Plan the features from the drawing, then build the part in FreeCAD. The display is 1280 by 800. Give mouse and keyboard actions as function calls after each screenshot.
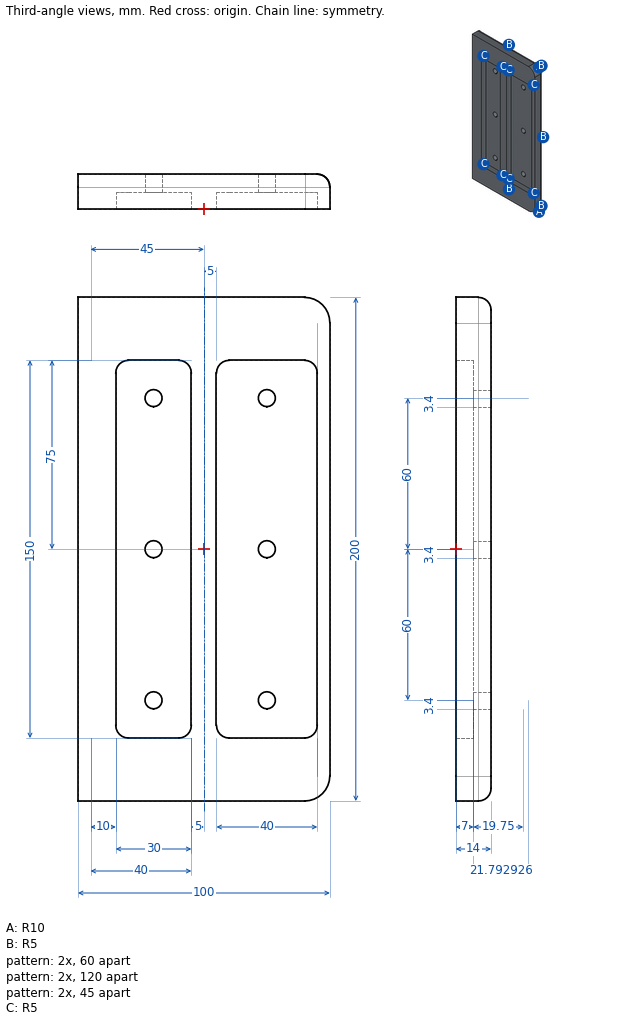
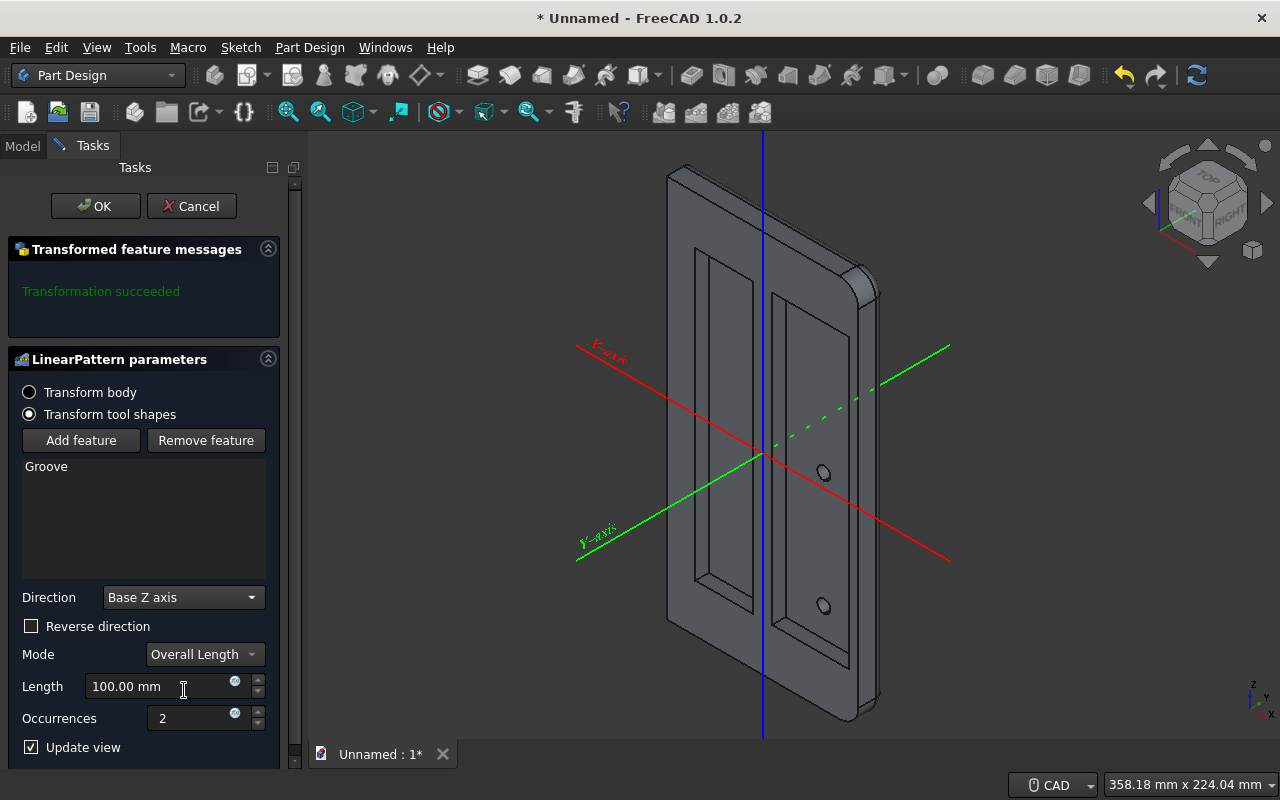
click(206, 654)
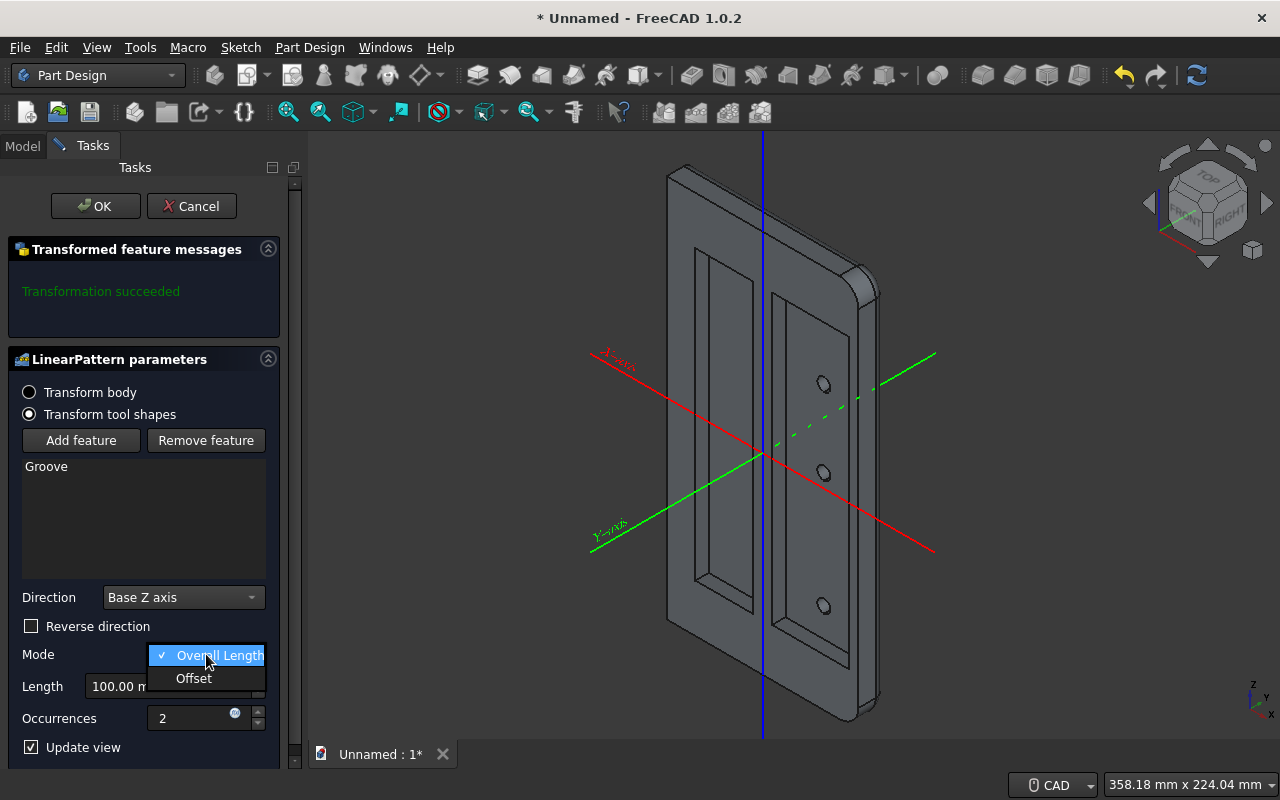
click(206, 678)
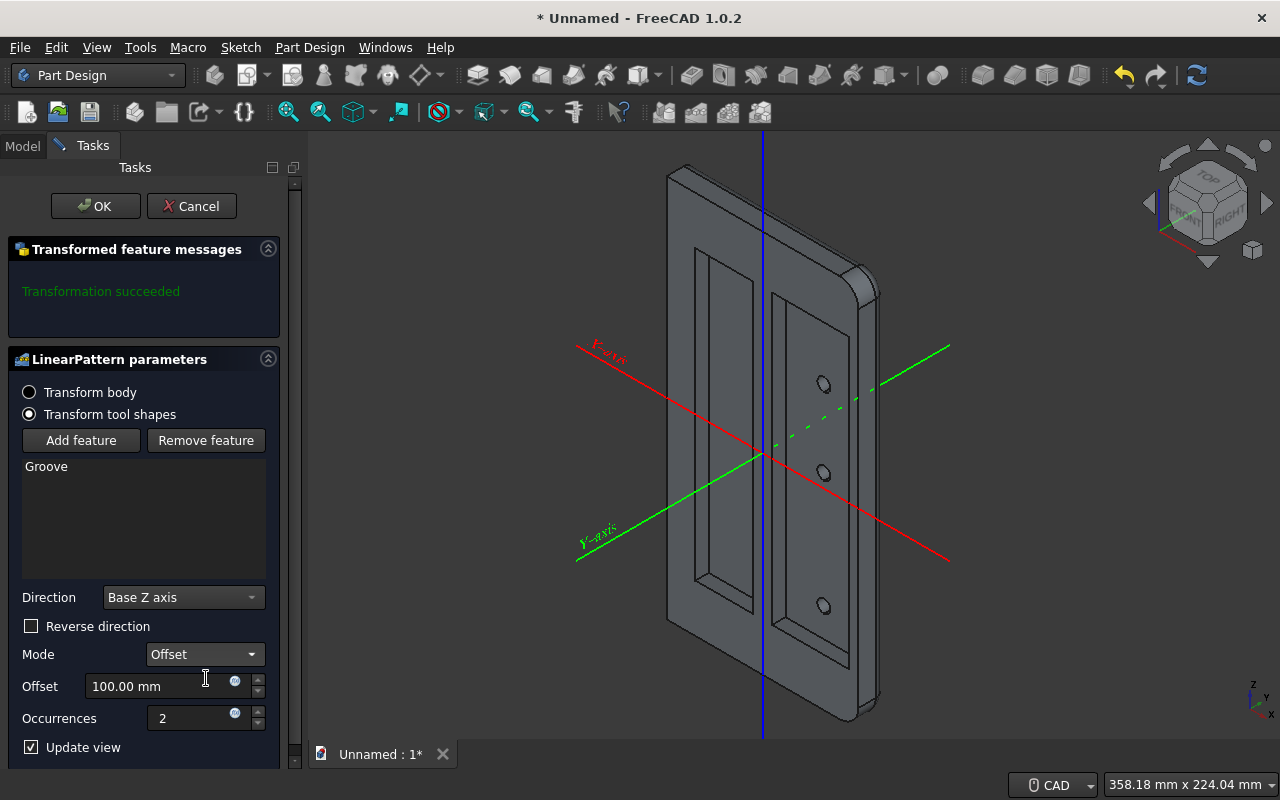
triple_click(168, 686)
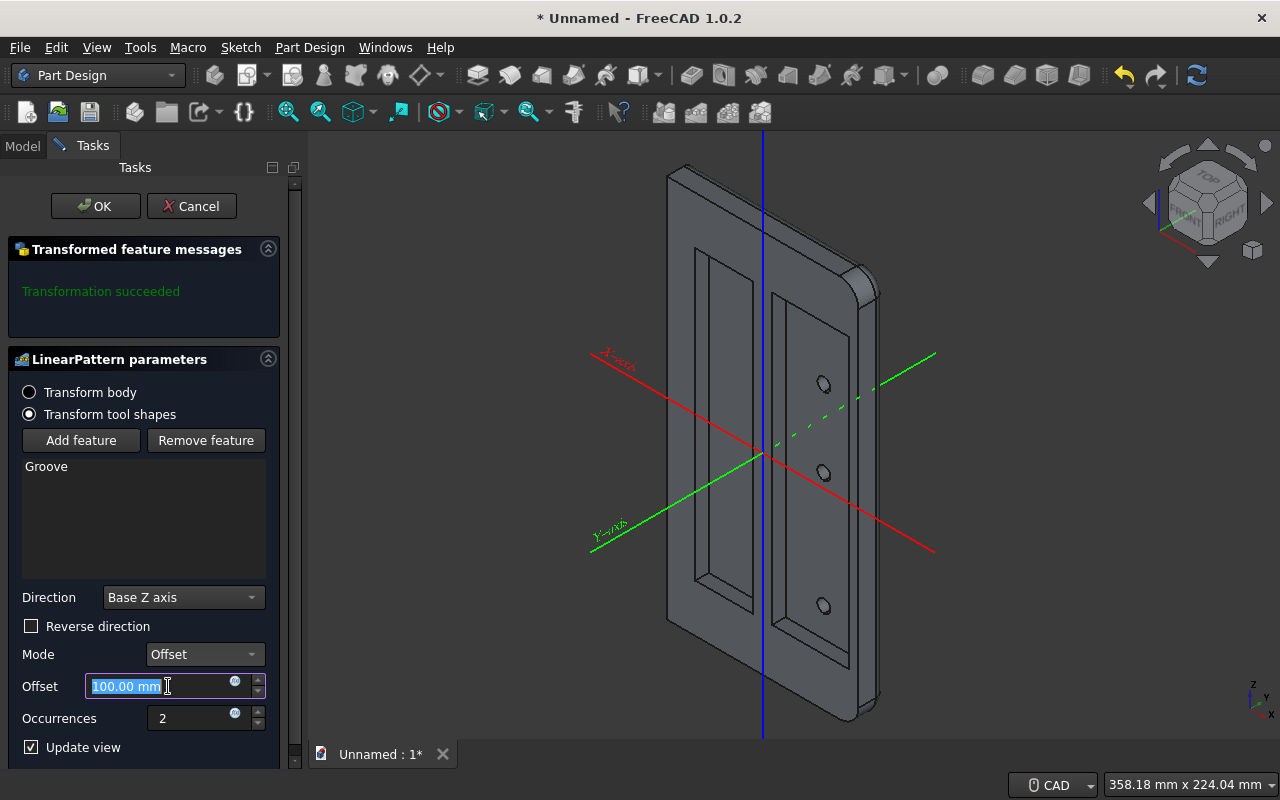
text(120)
key(Tab)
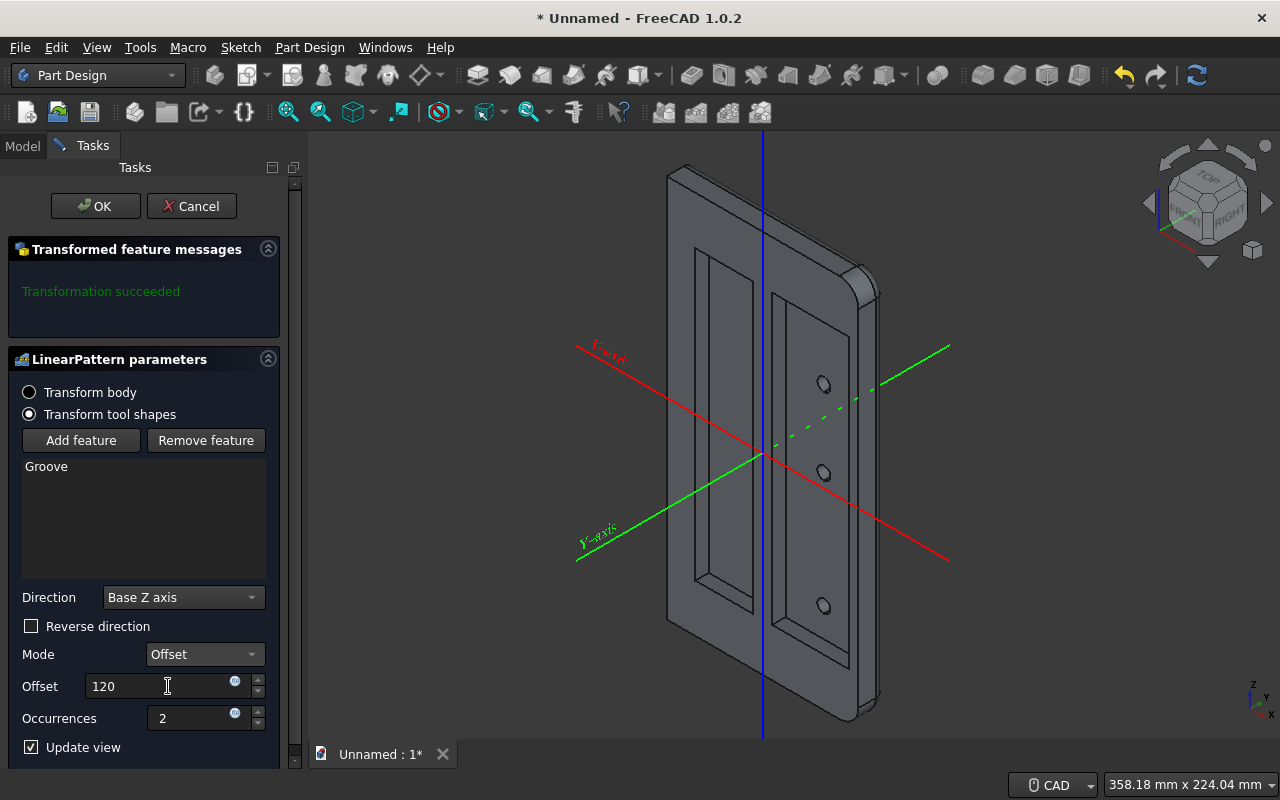
triple_click(198, 718)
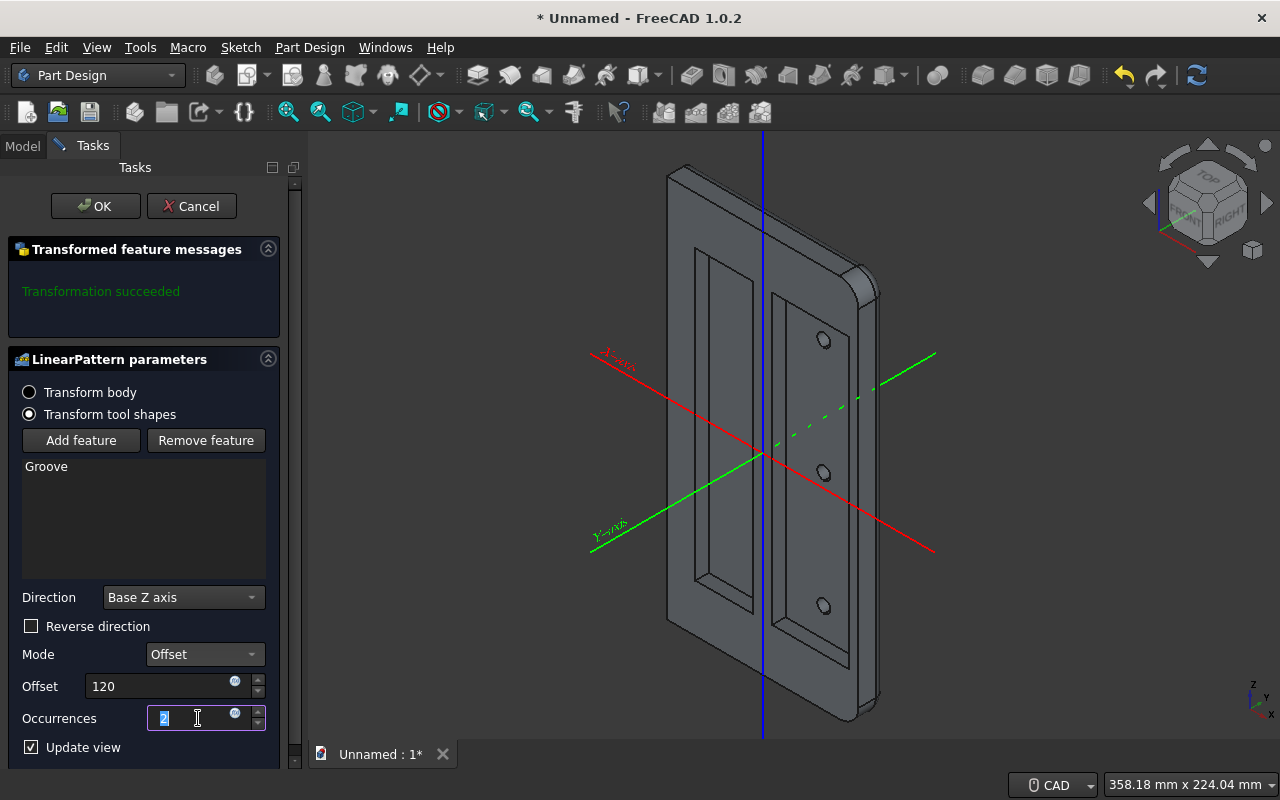
text(2)
key(Tab)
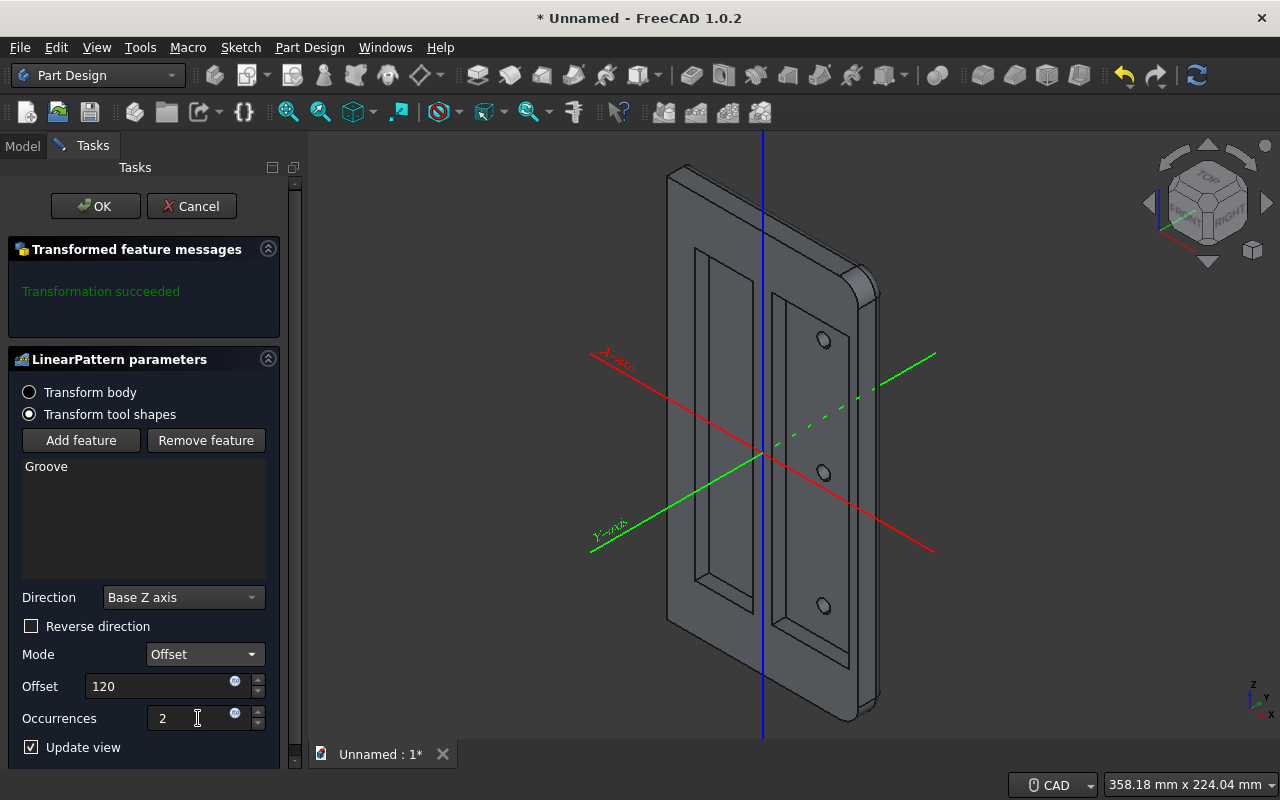
click(96, 206)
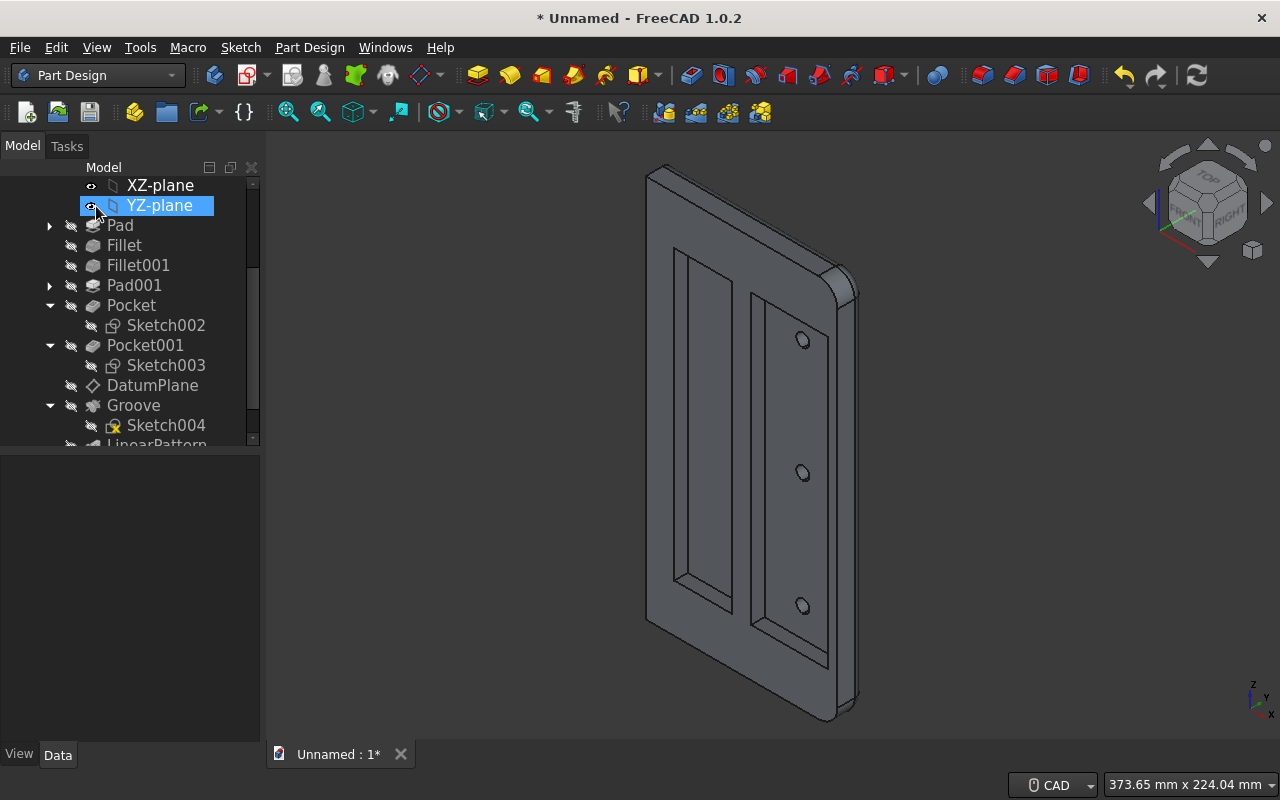
click(116, 406)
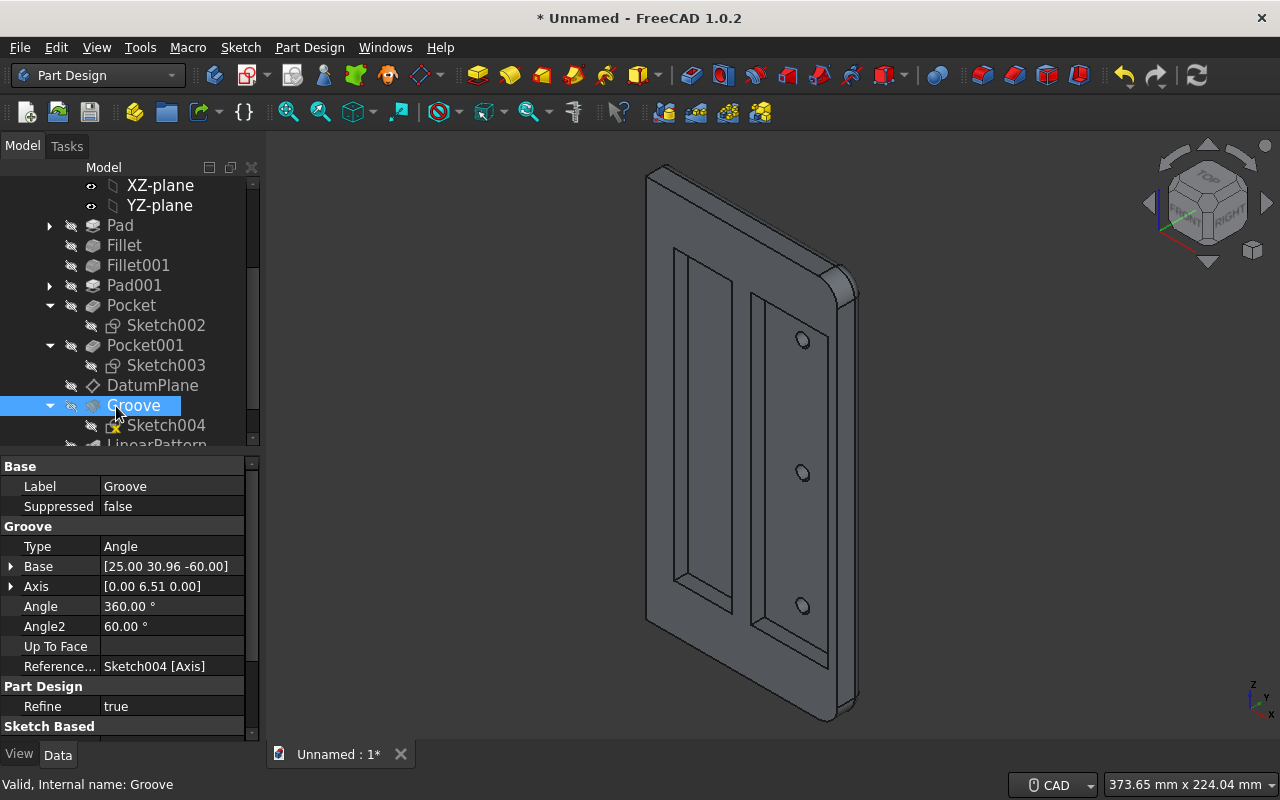
click(696, 112)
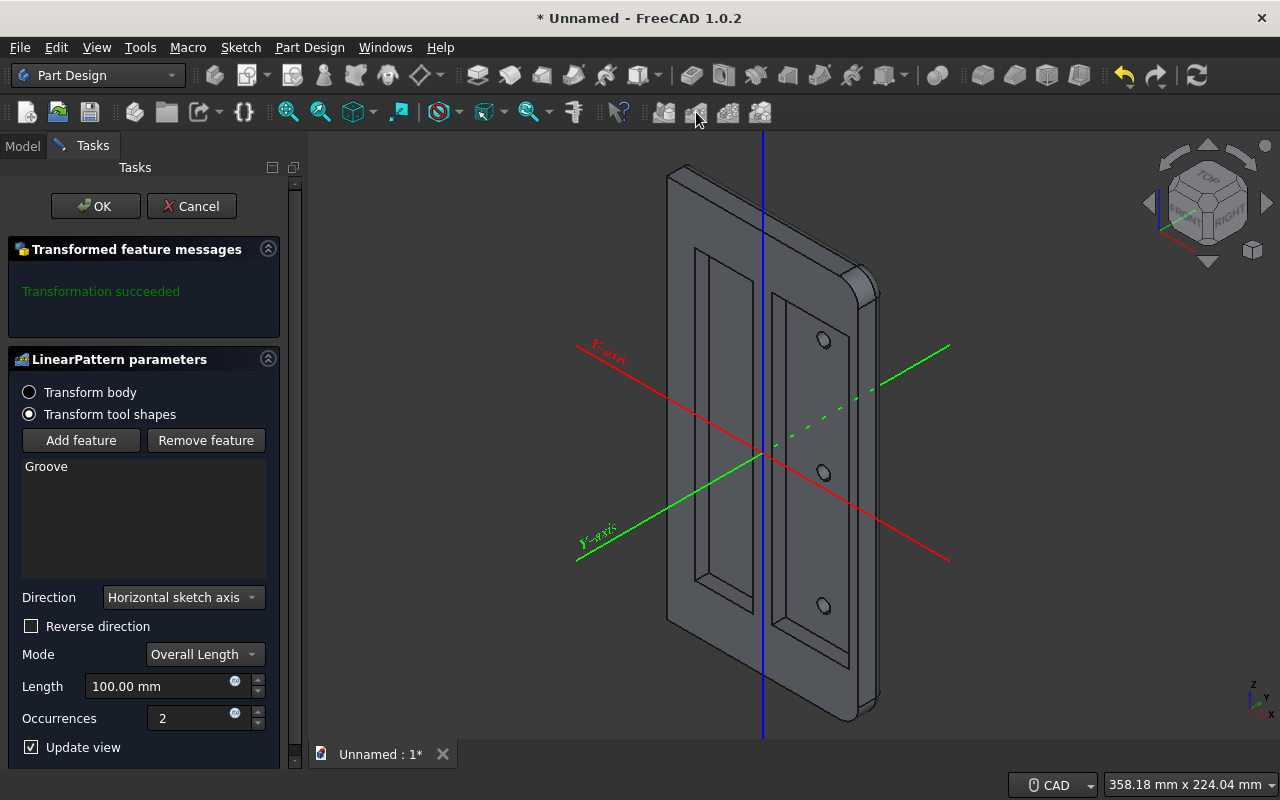
click(184, 598)